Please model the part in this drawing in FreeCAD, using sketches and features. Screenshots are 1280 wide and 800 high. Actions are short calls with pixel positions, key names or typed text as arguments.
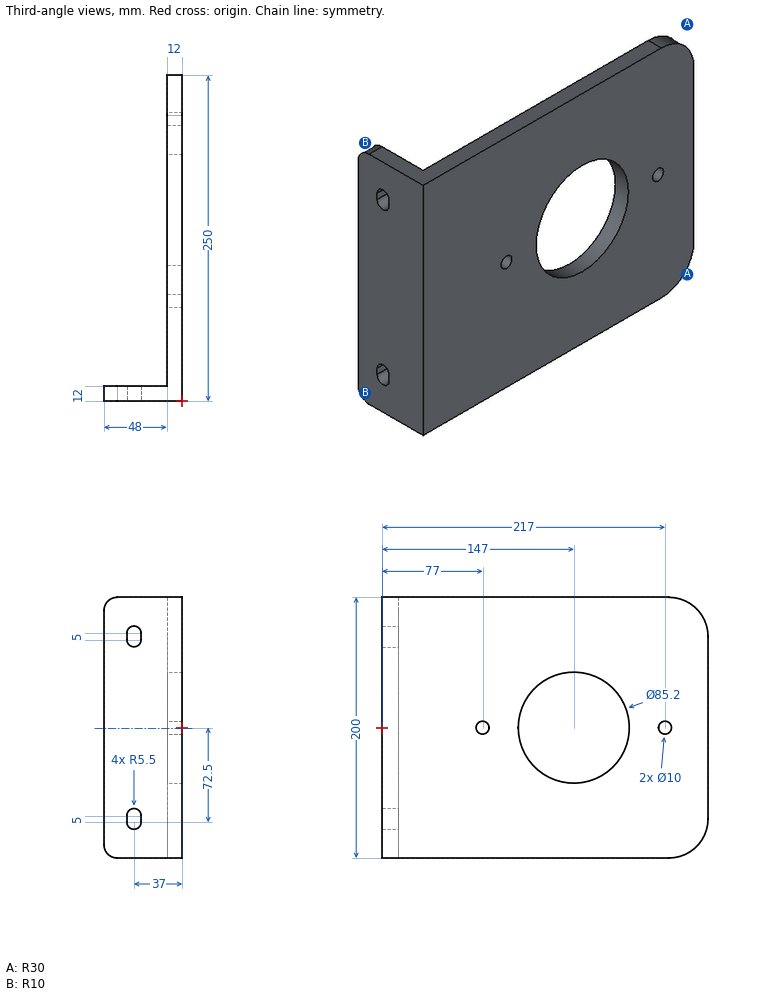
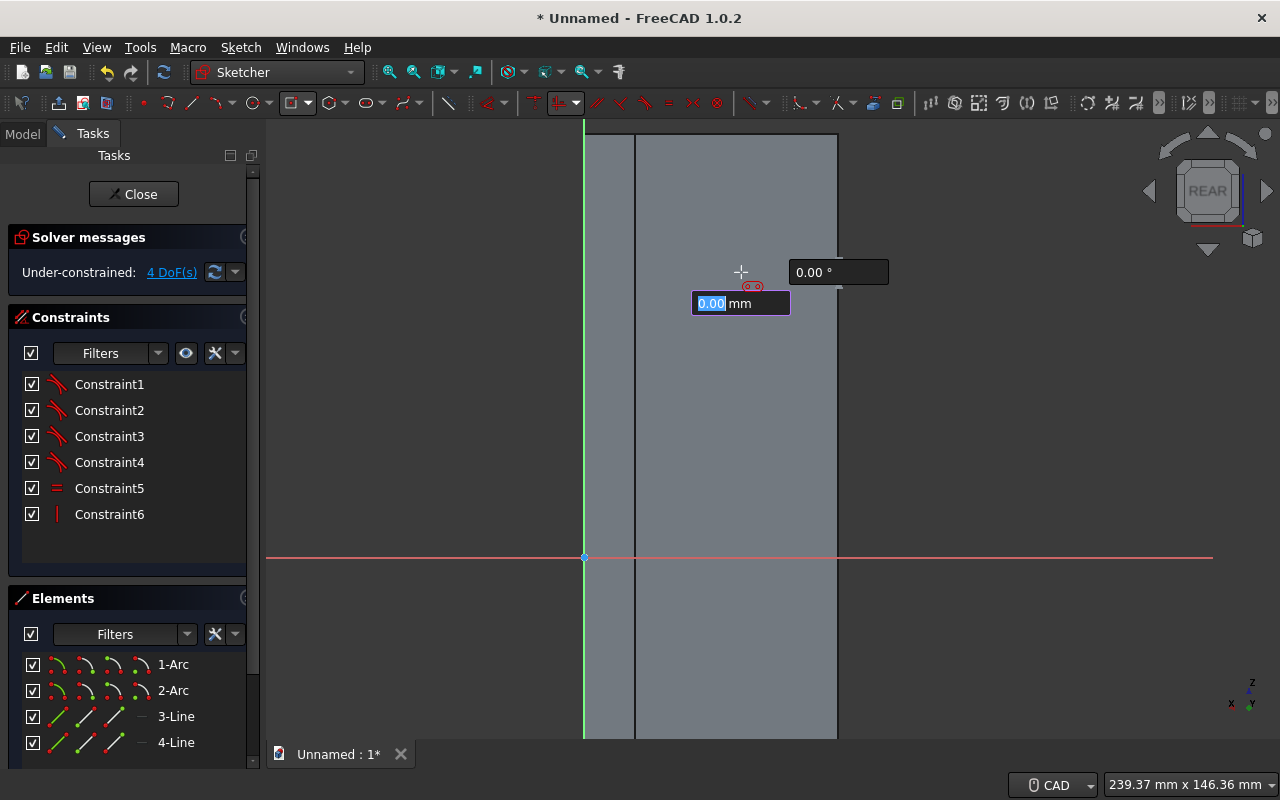
click(741, 251)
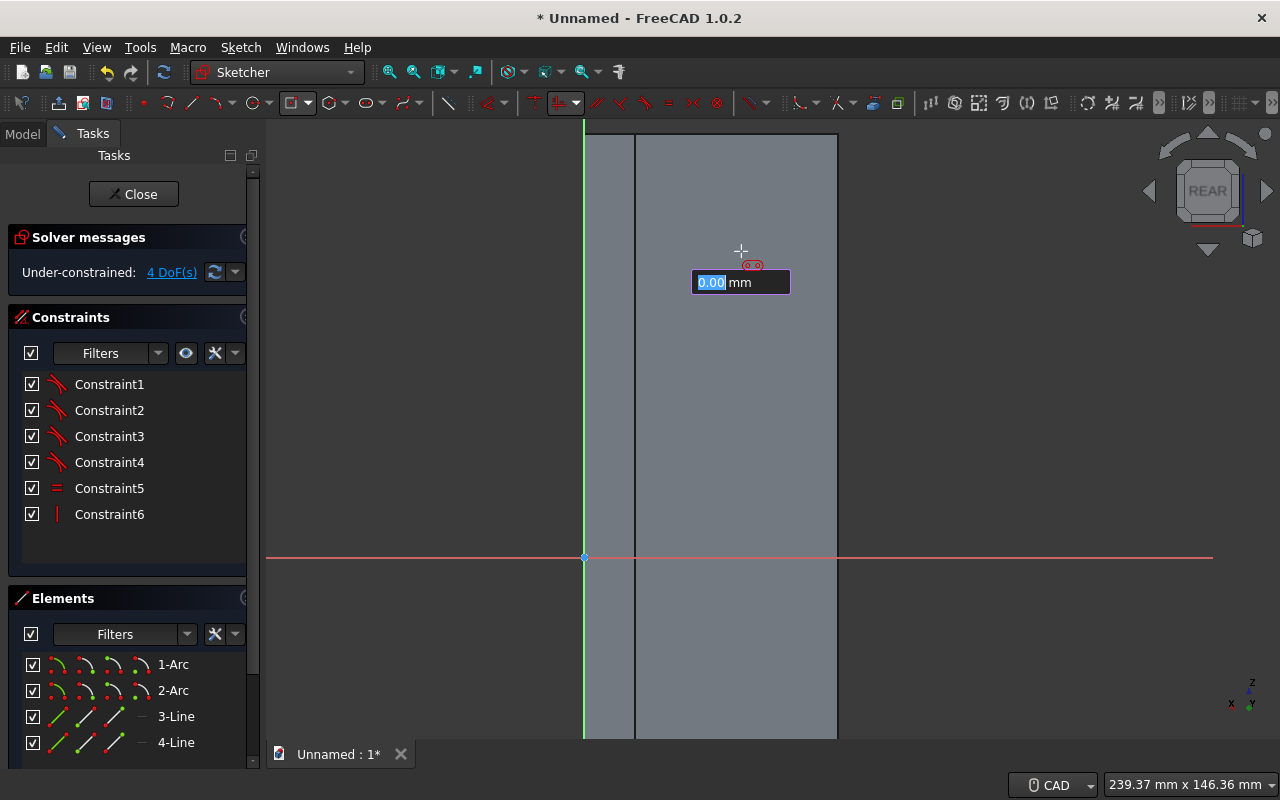
click(764, 261)
key(Escape)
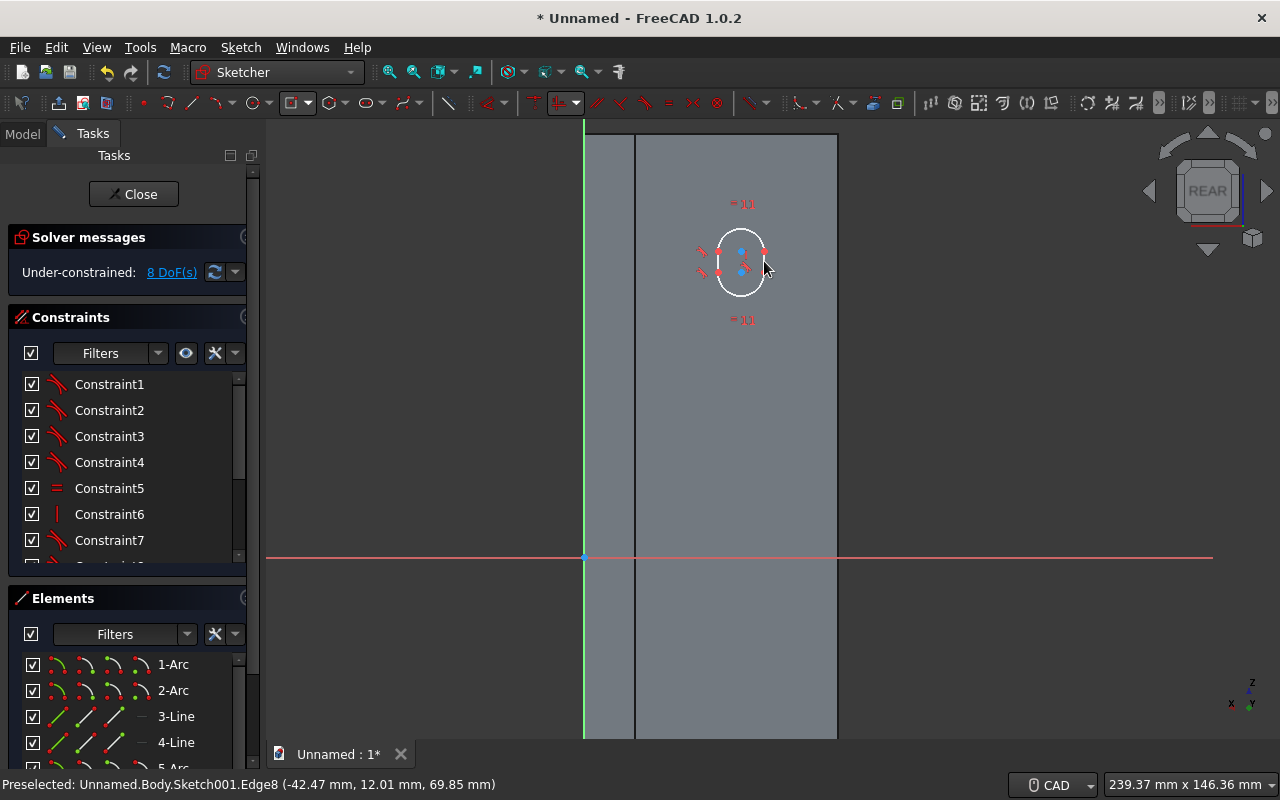
scroll(741, 272, down, 3)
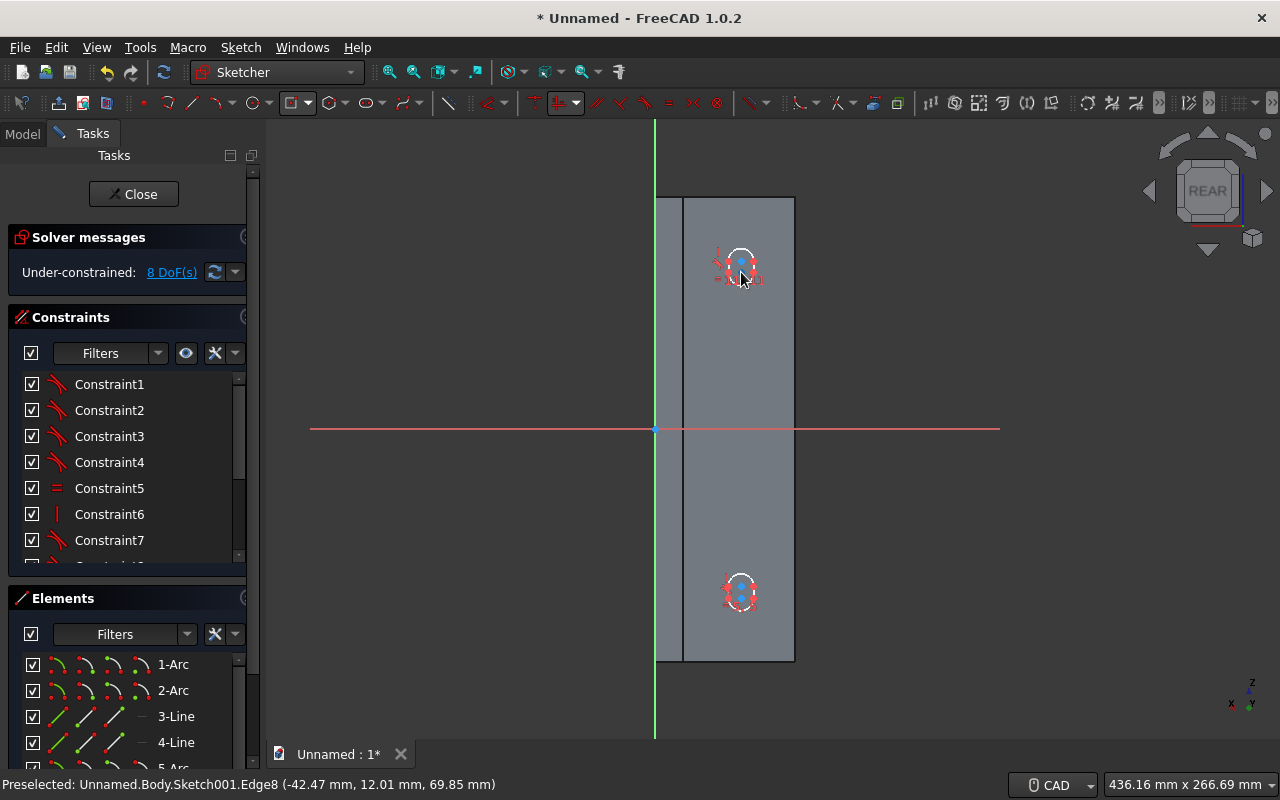
scroll(734, 608, up, 4)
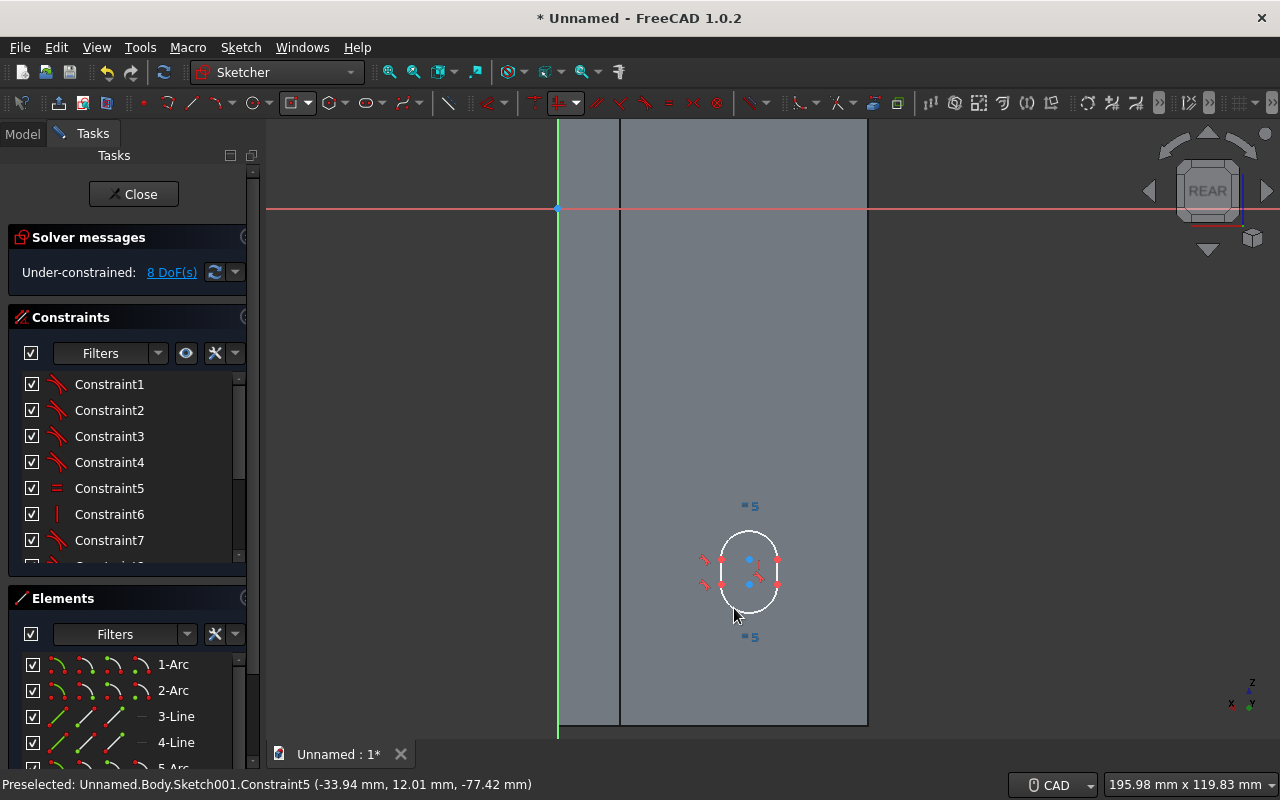
click(733, 608)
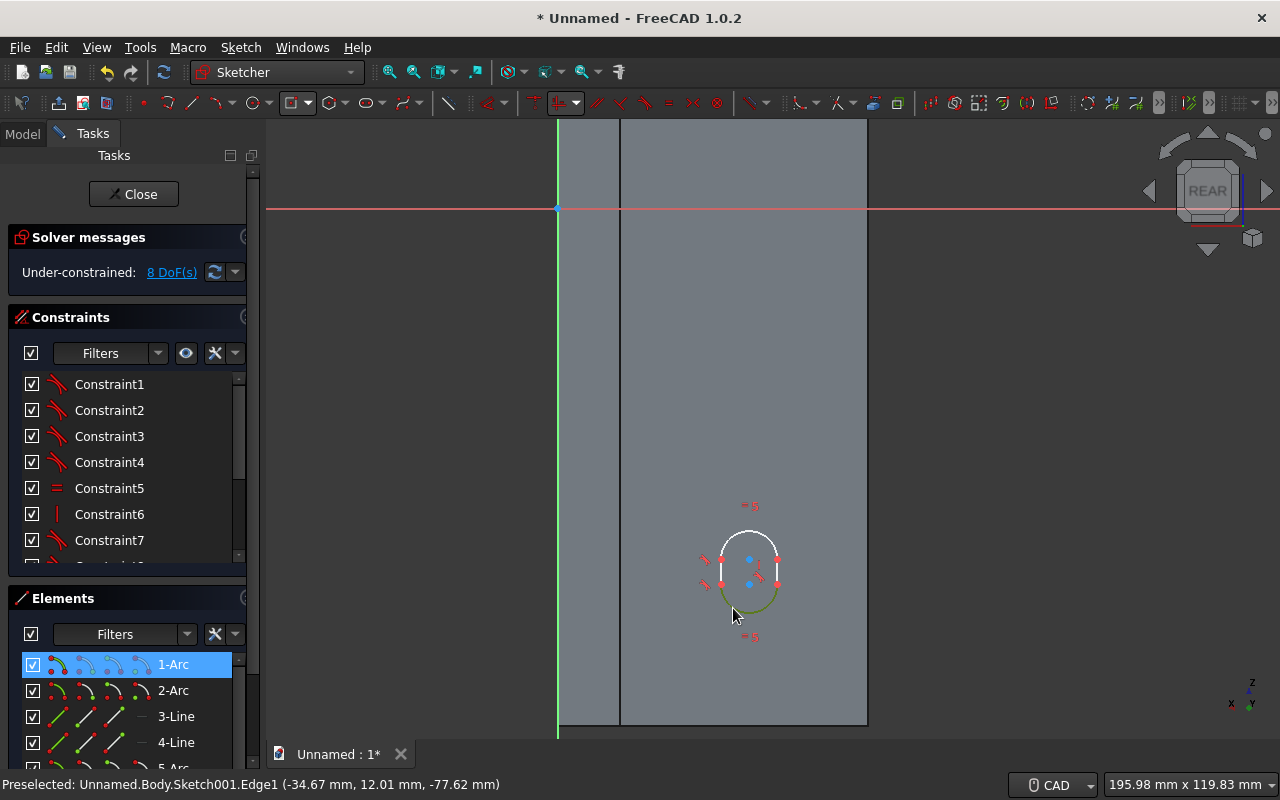
scroll(734, 609, down, 4)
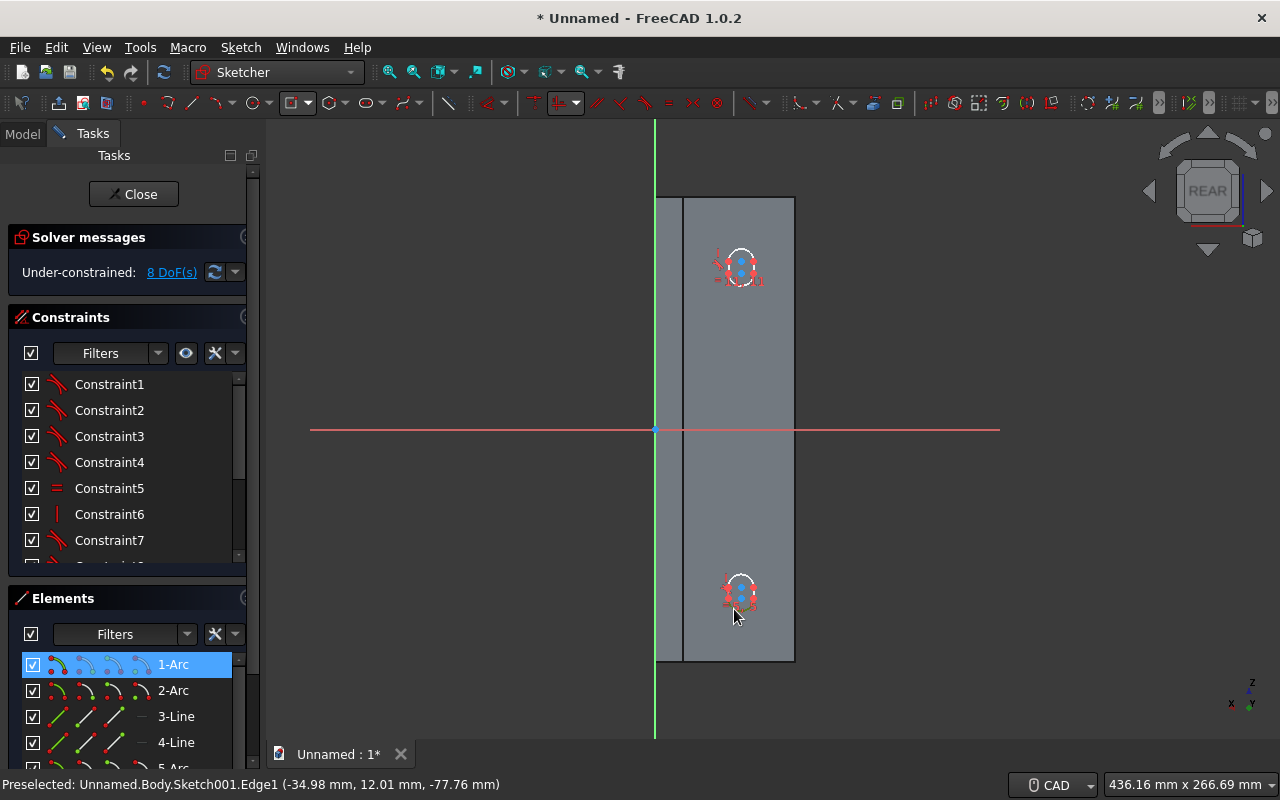
scroll(734, 283, up, 4)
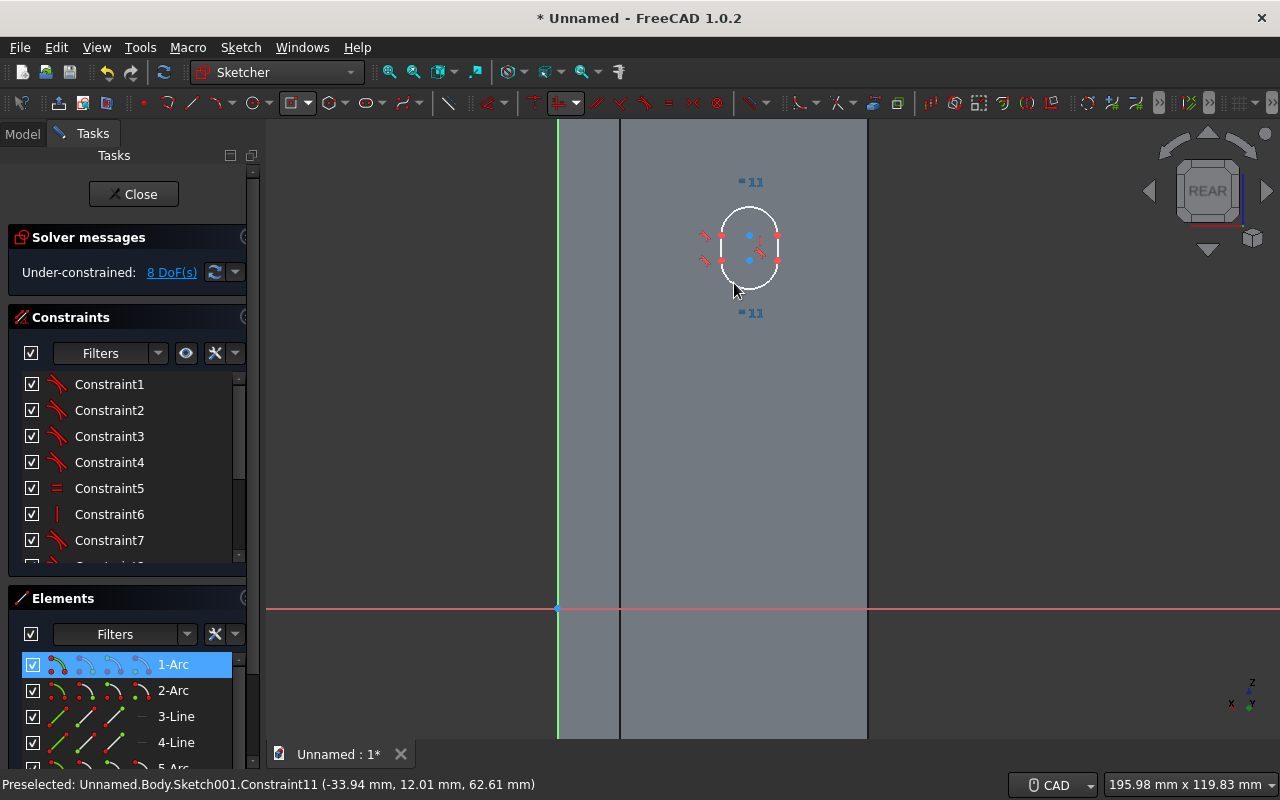
click(733, 284)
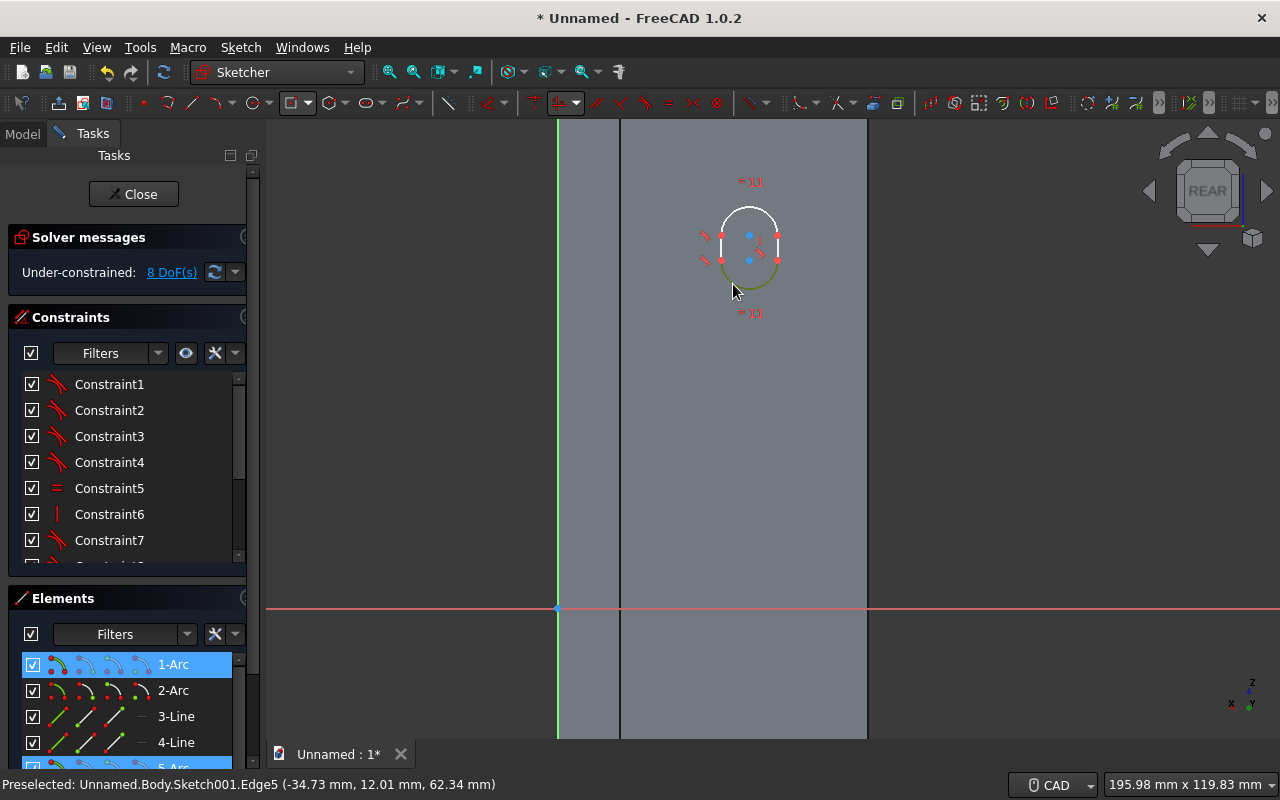
key(e)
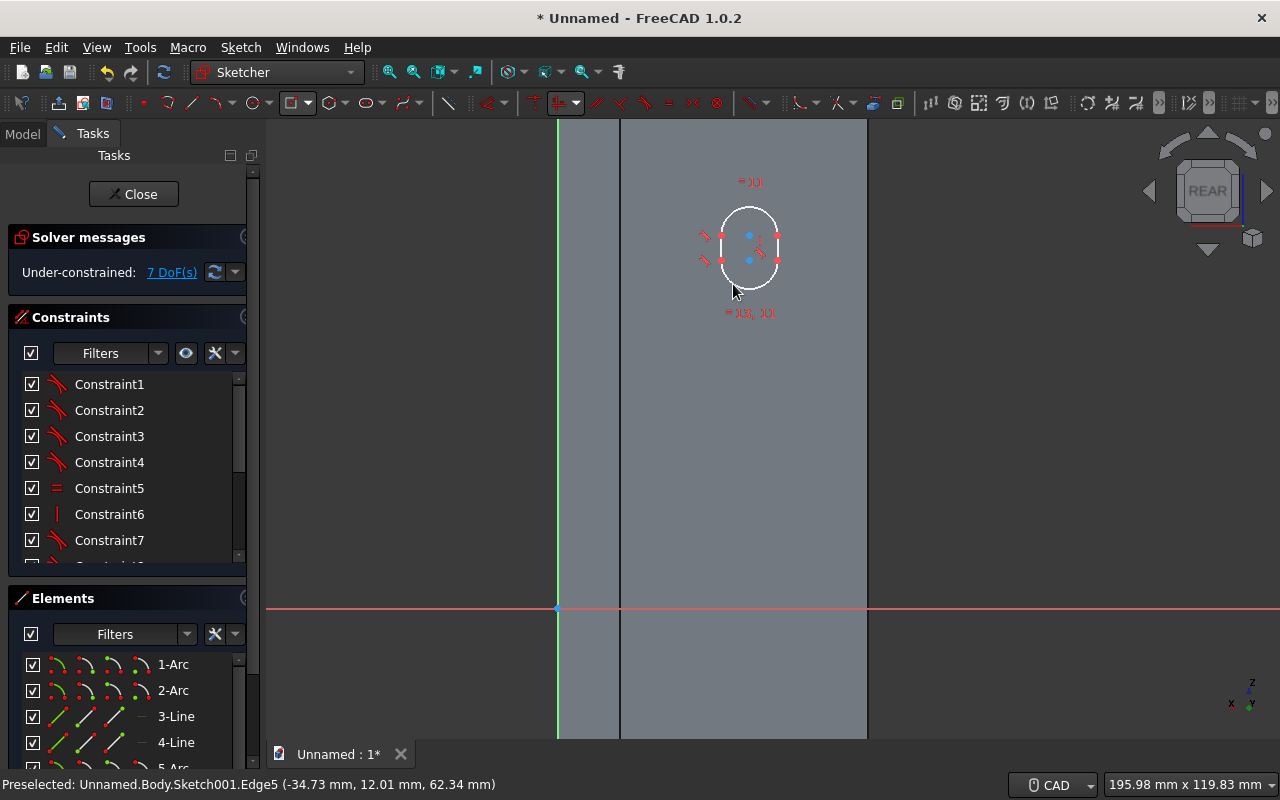
scroll(734, 282, down, 4)